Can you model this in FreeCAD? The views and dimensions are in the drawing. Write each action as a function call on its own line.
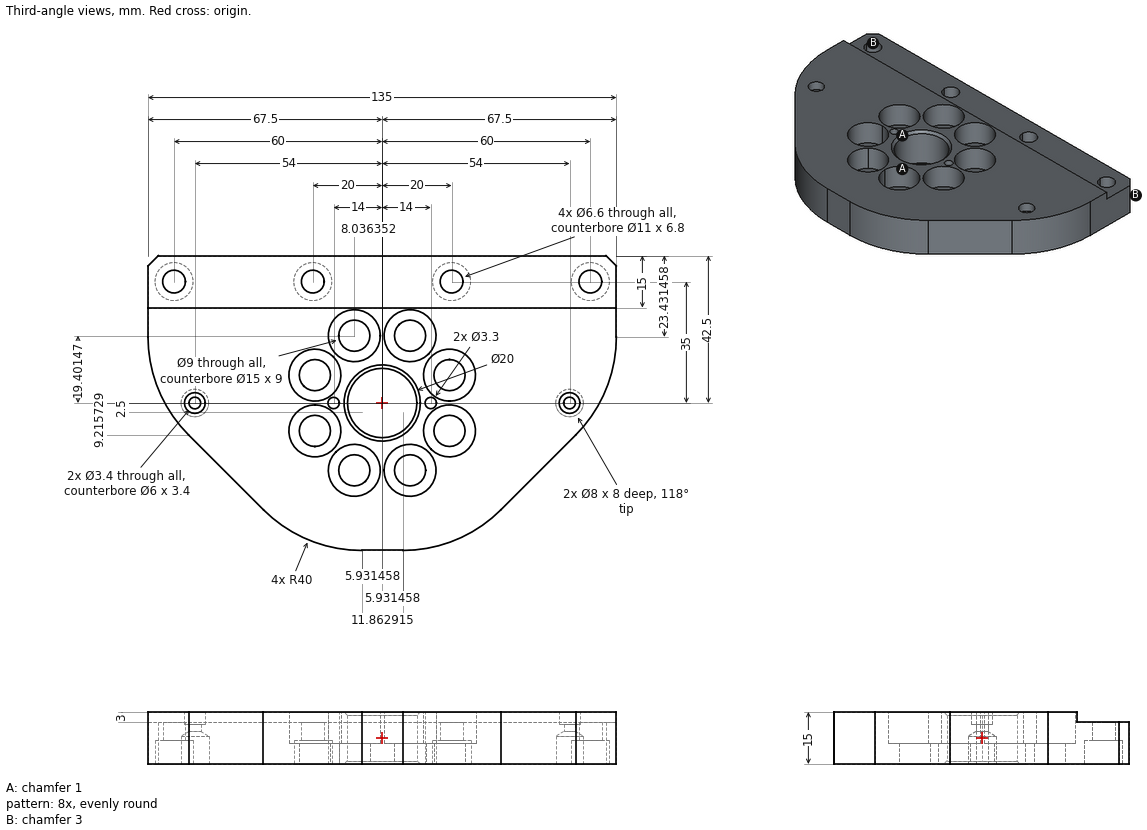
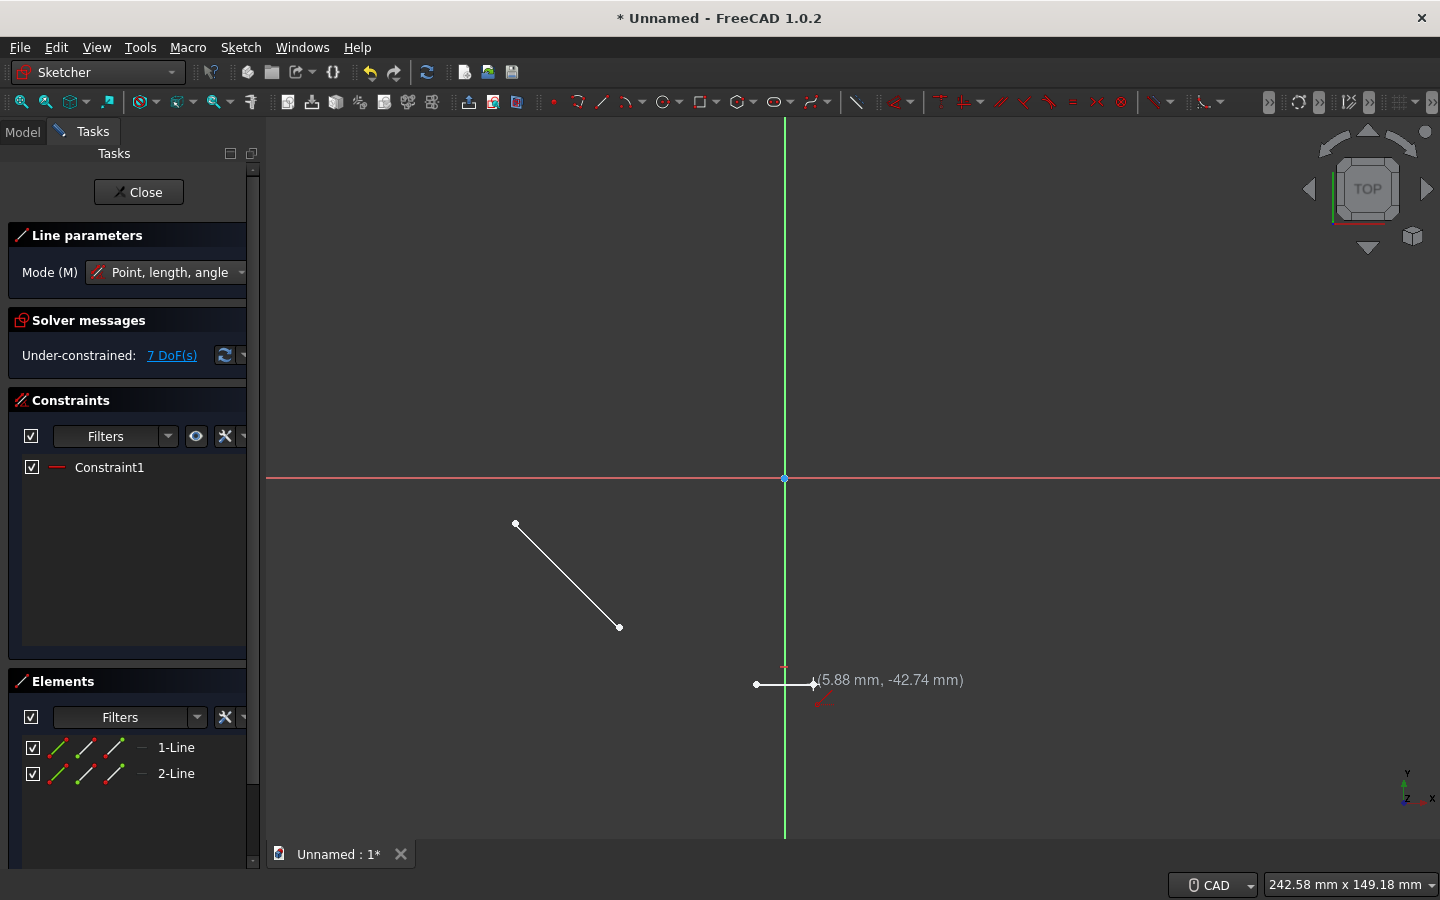
click(950, 627)
click(1055, 523)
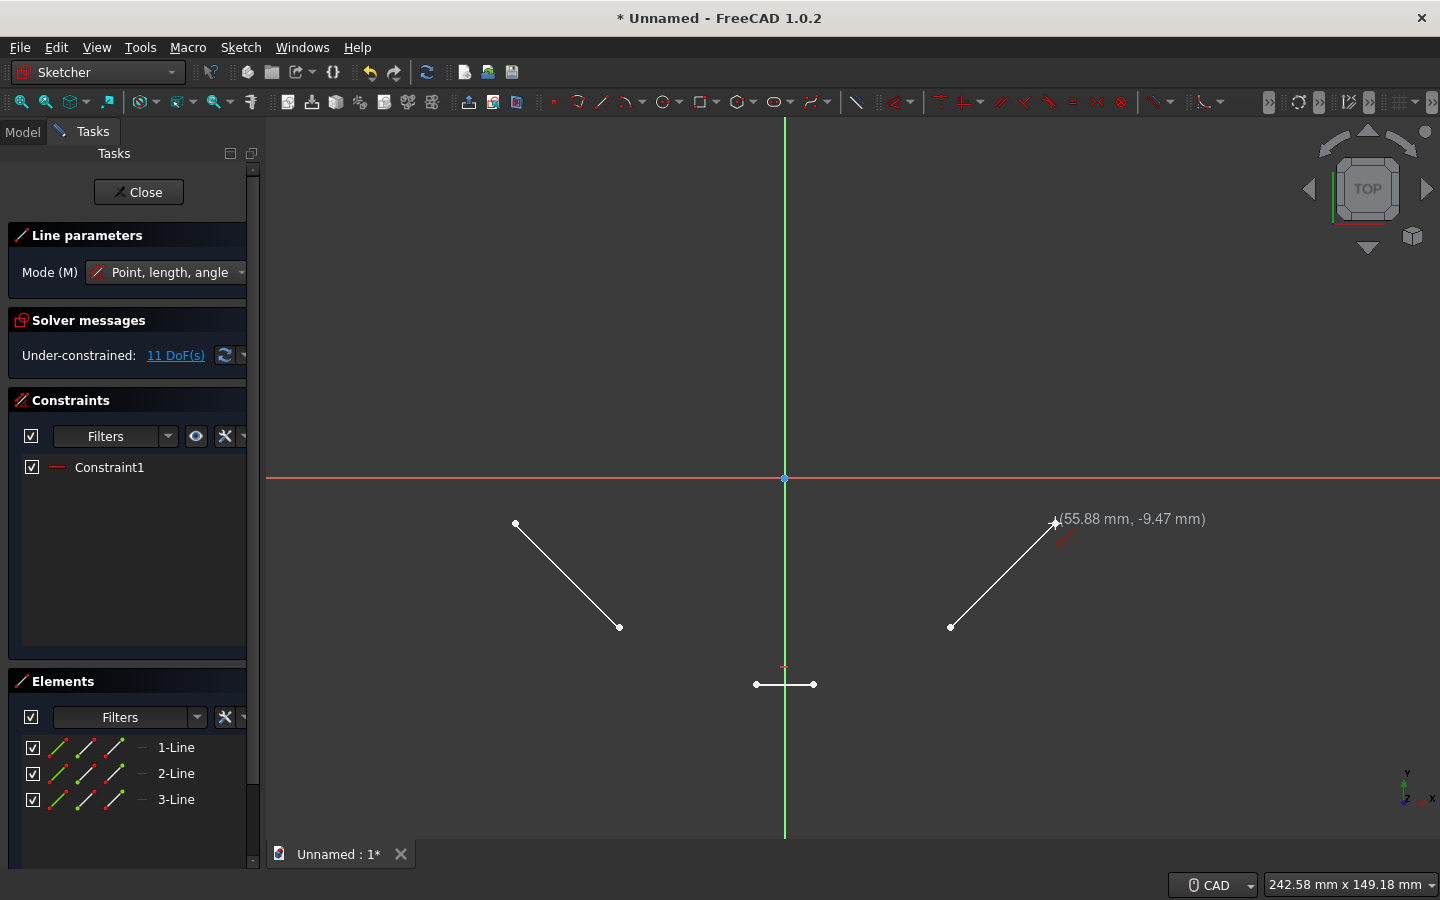
click(578, 102)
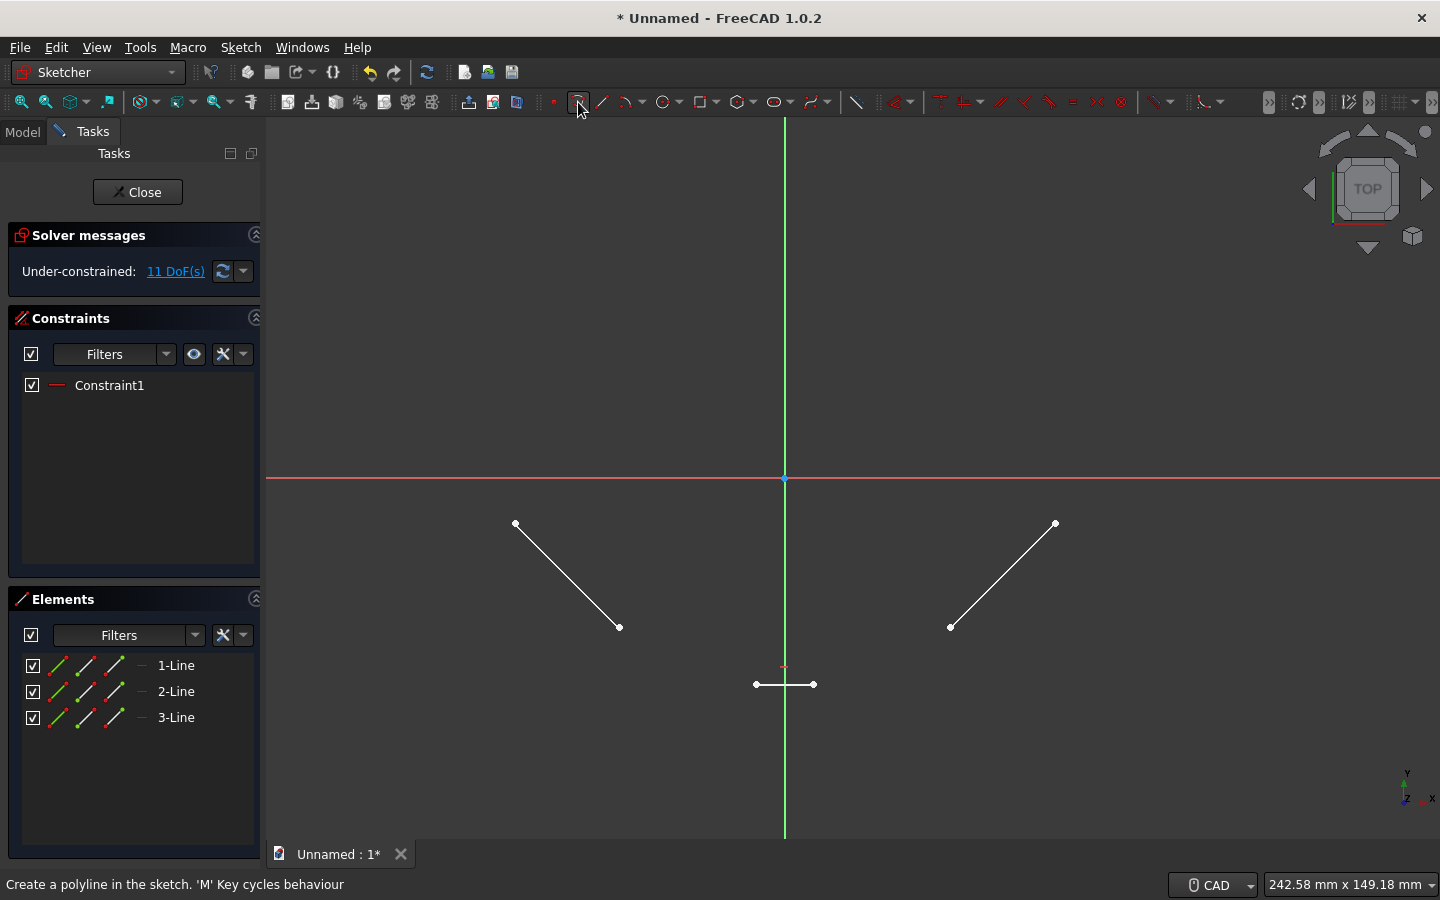
click(1111, 386)
click(1111, 272)
click(458, 272)
click(458, 386)
right_click(458, 386)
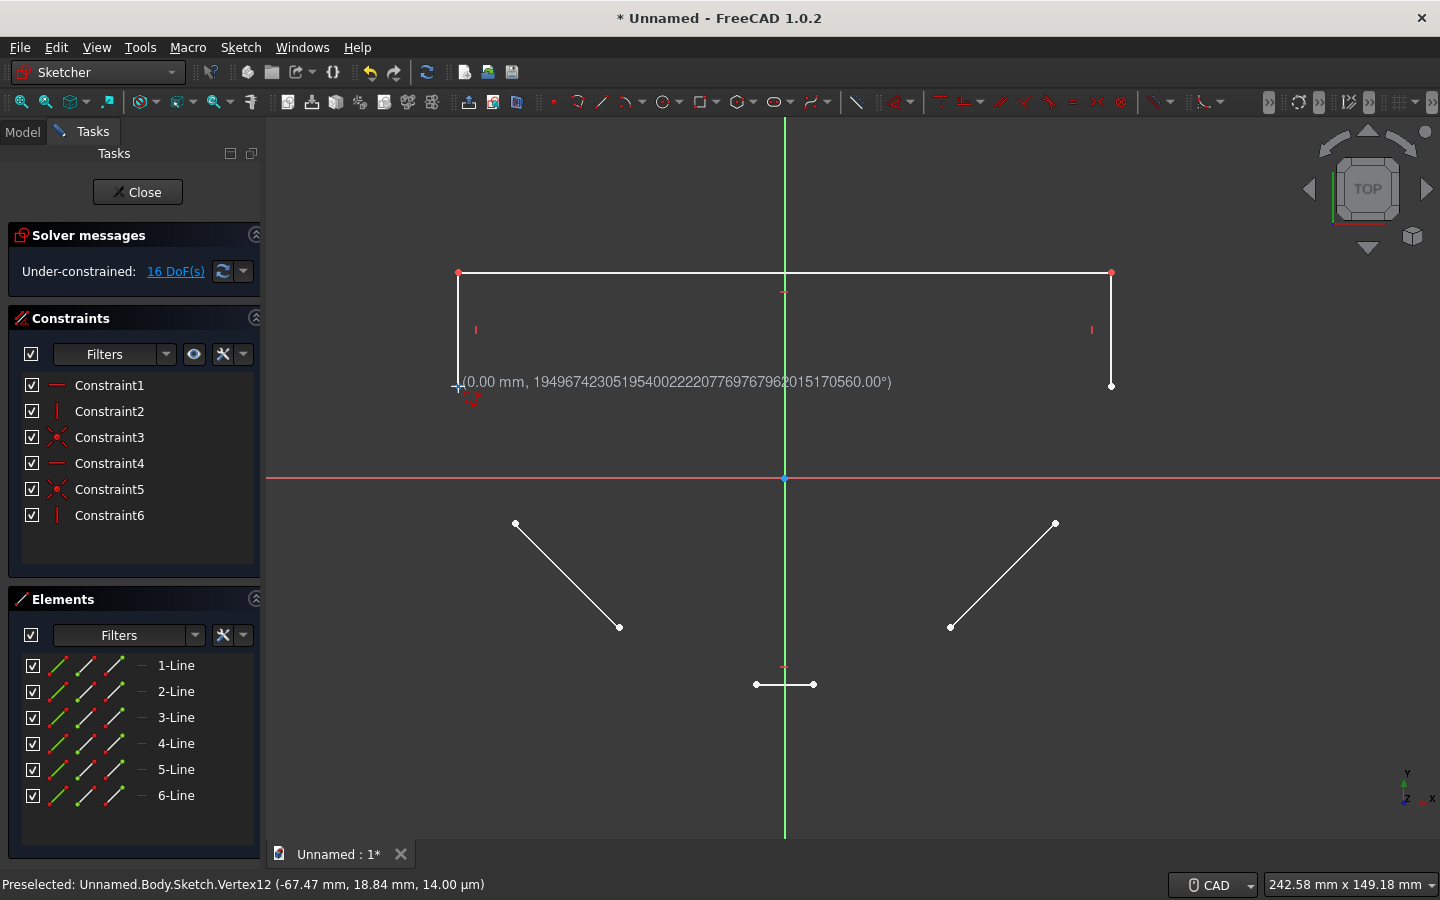
click(644, 102)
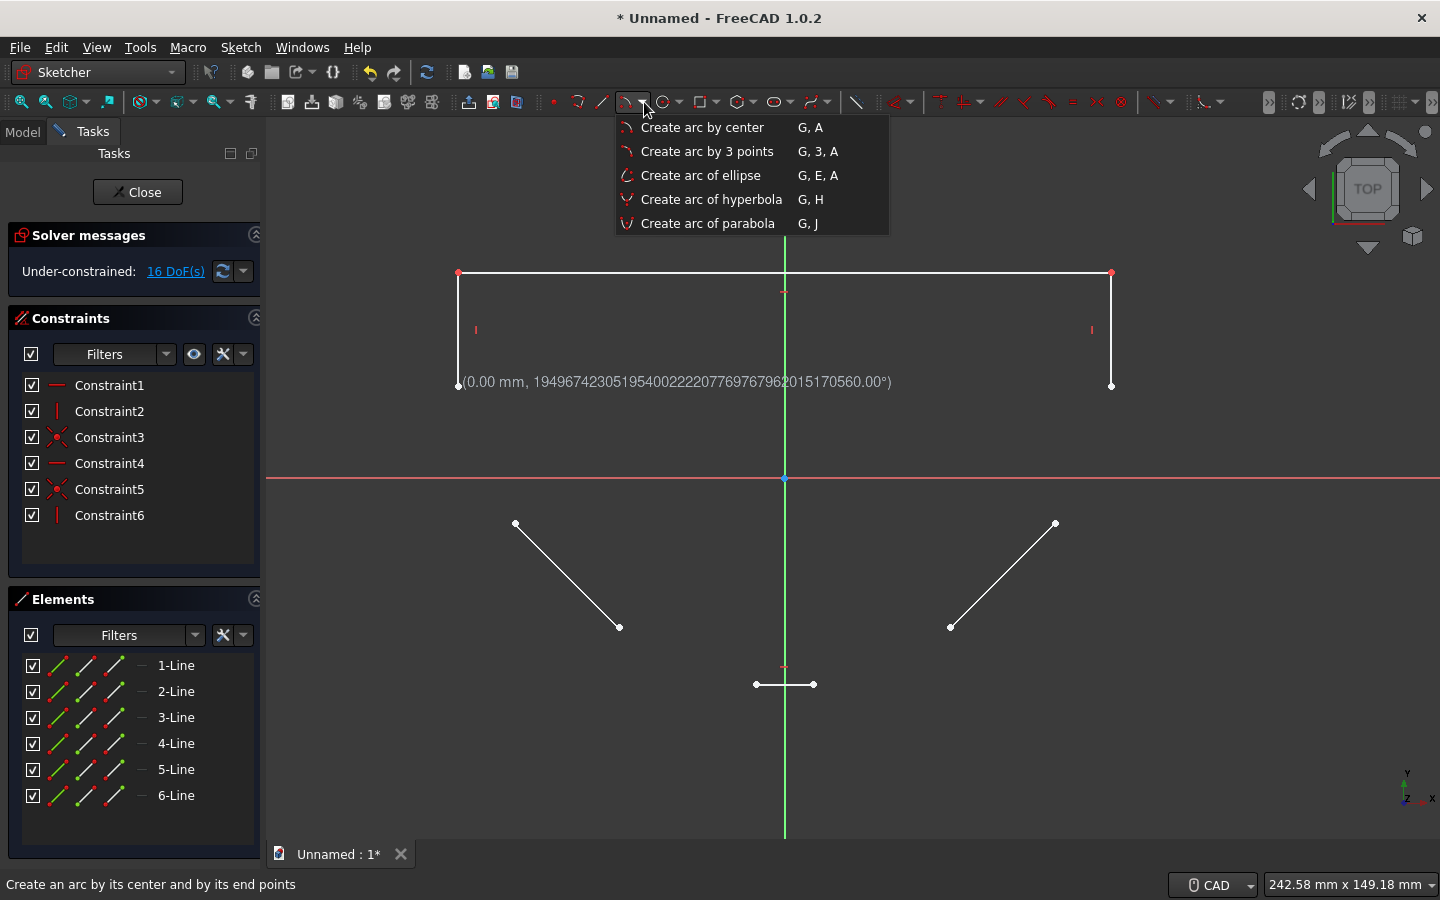
click(752, 151)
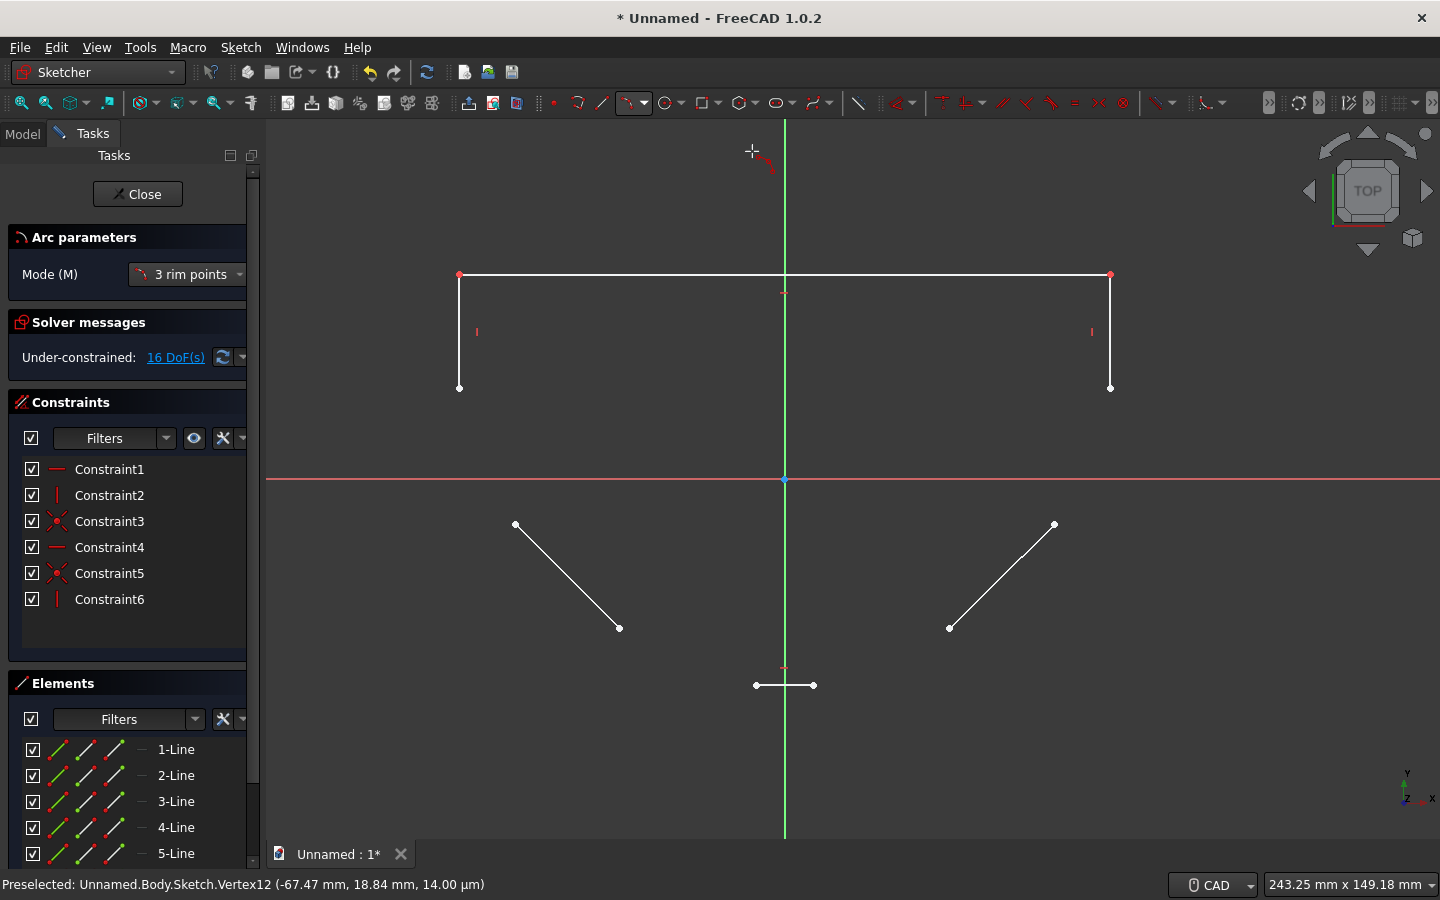
click(620, 629)
click(756, 685)
click(682, 670)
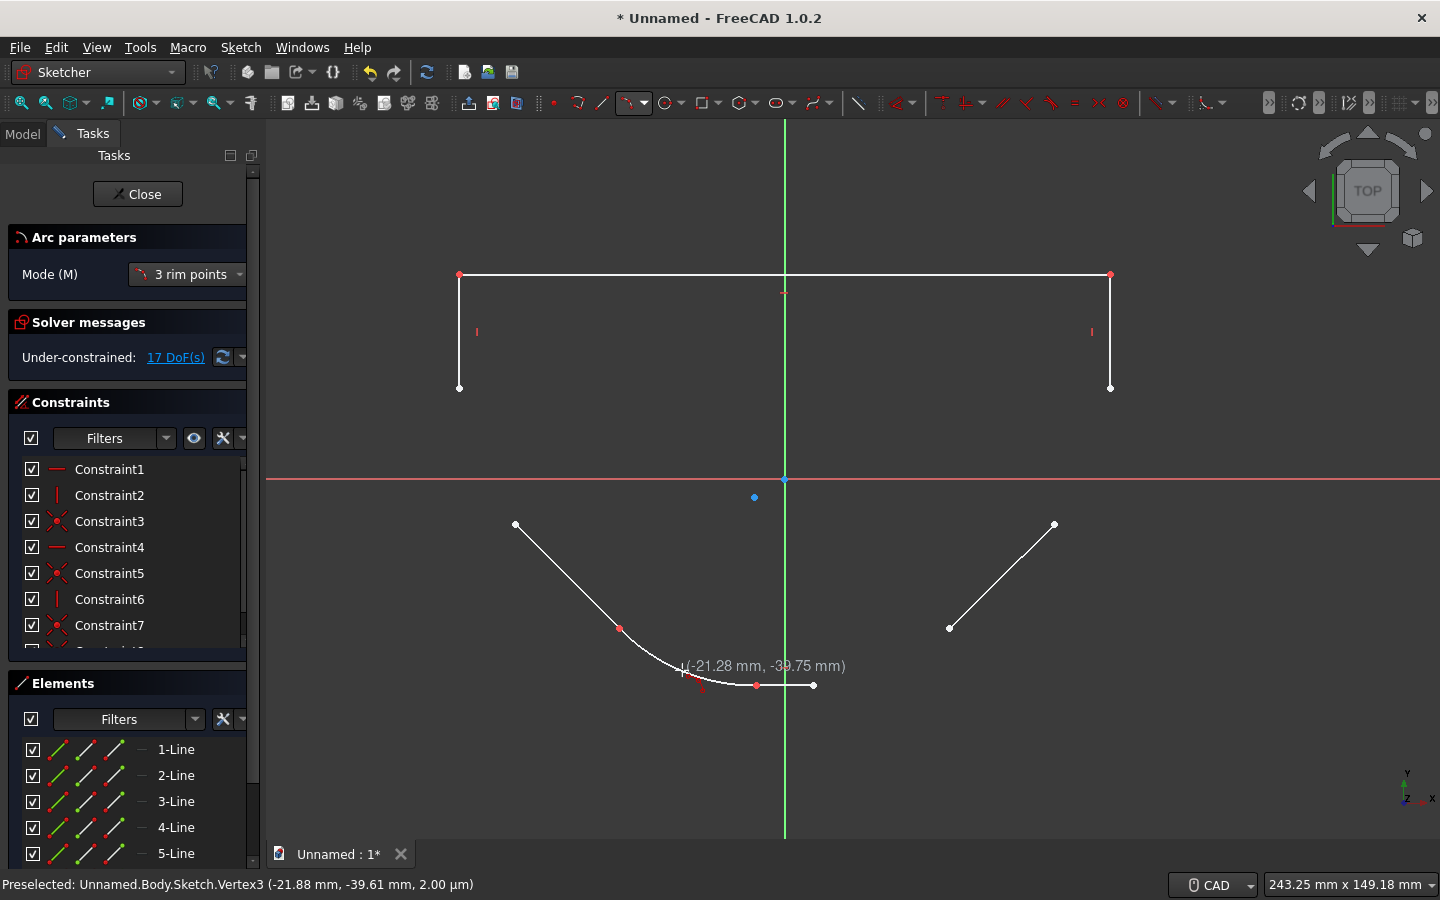
click(813, 685)
click(950, 629)
click(887, 670)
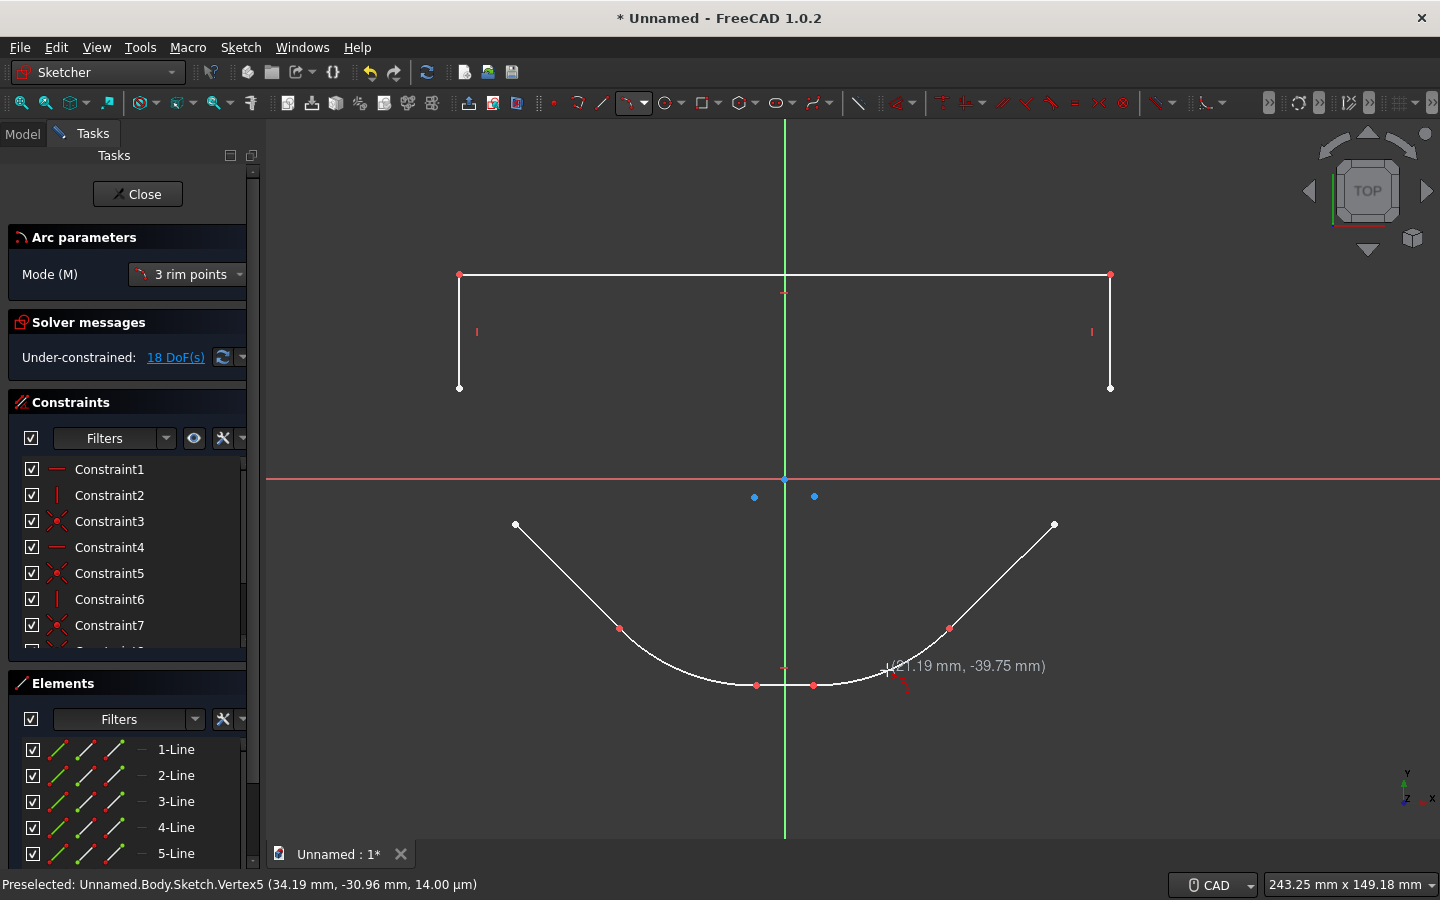
click(1054, 525)
click(1110, 388)
click(1096, 461)